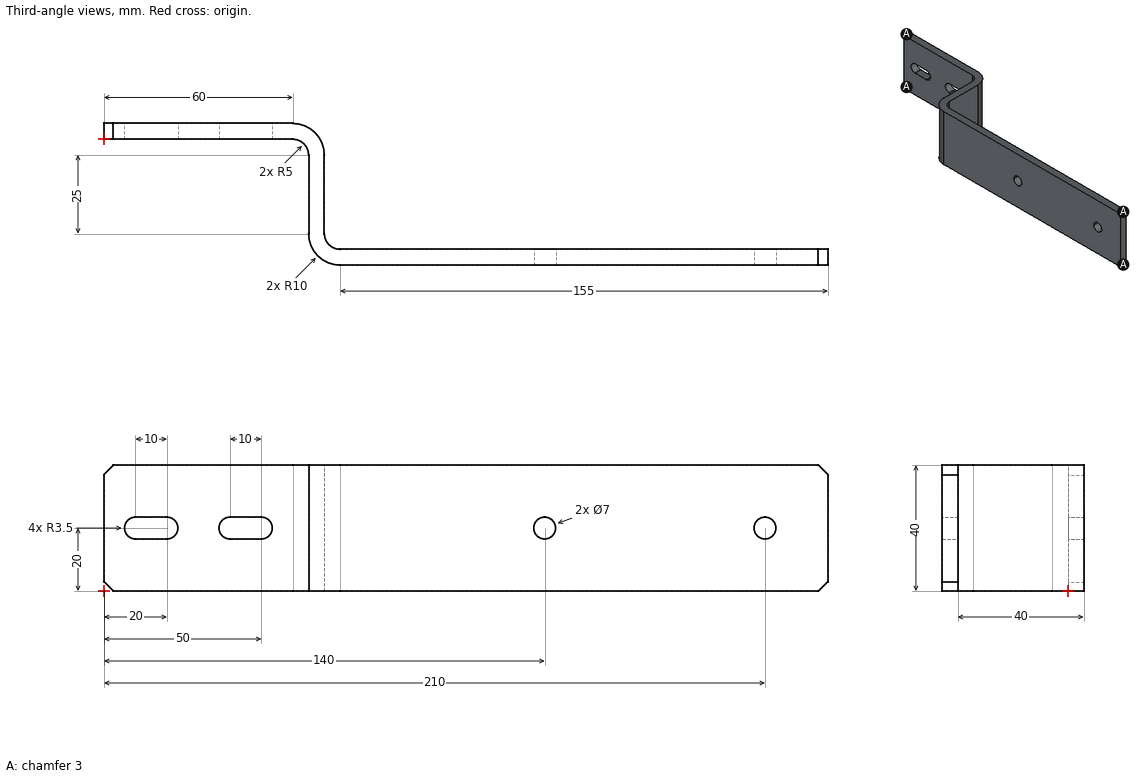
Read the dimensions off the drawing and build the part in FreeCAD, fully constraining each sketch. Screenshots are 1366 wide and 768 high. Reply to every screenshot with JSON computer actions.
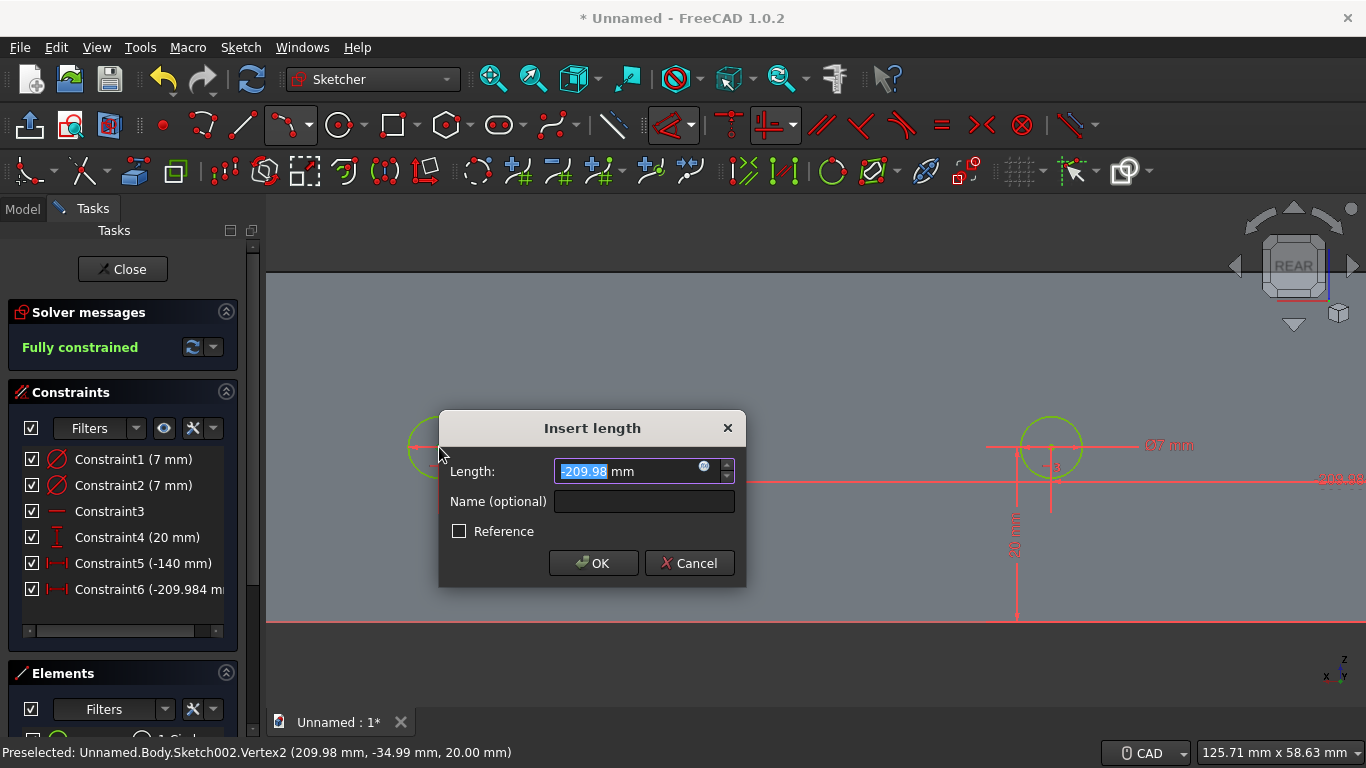
{"action": "type", "text": "-210"}
{"action": "key", "text": "Return"}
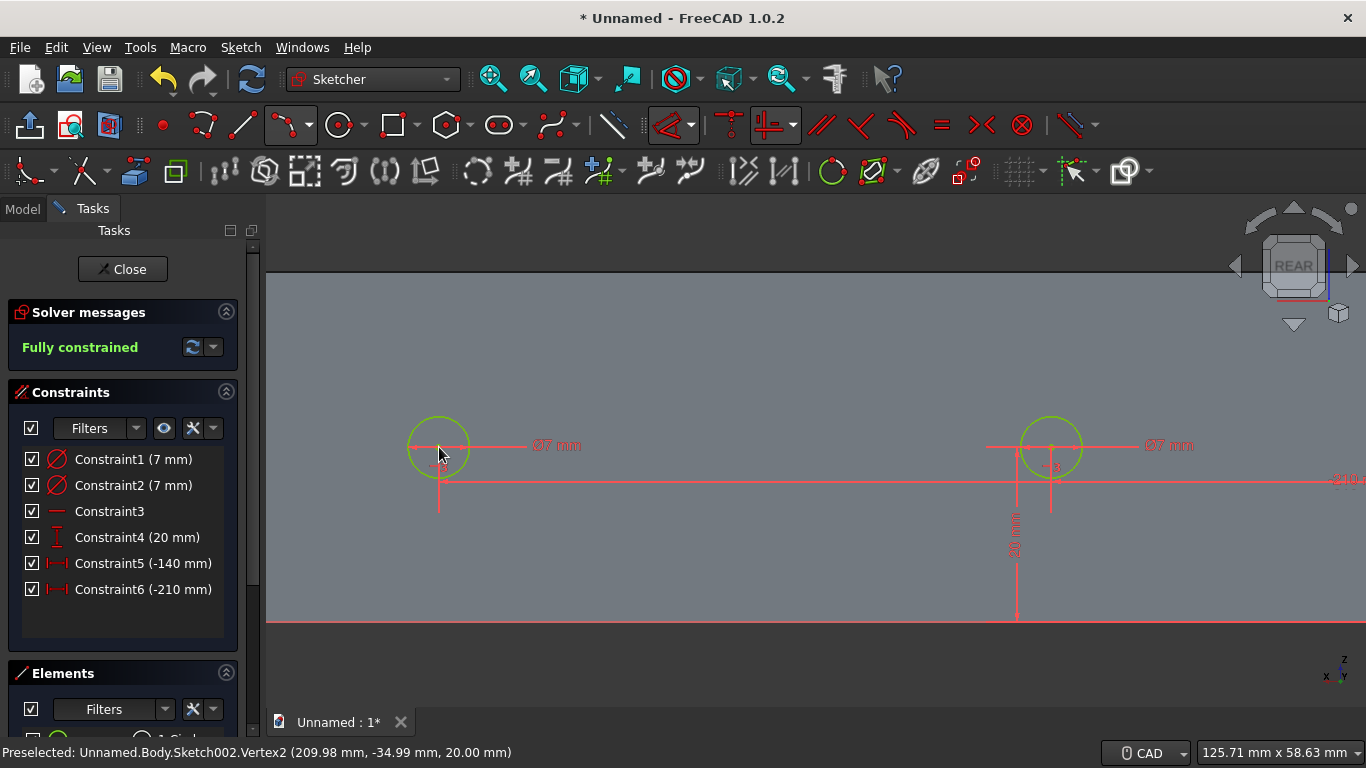
{"action": "left_click", "coordinate": [123, 269]}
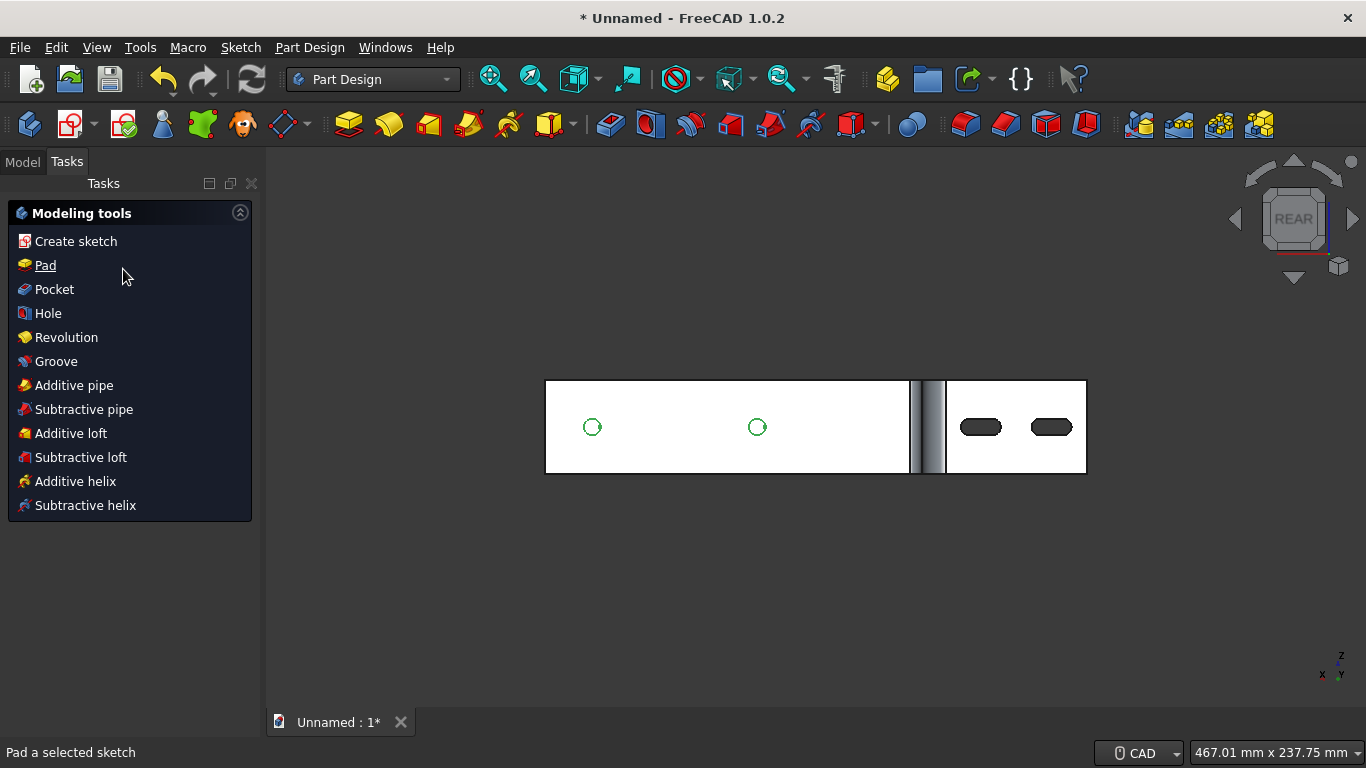
{"action": "left_click", "coordinate": [612, 124]}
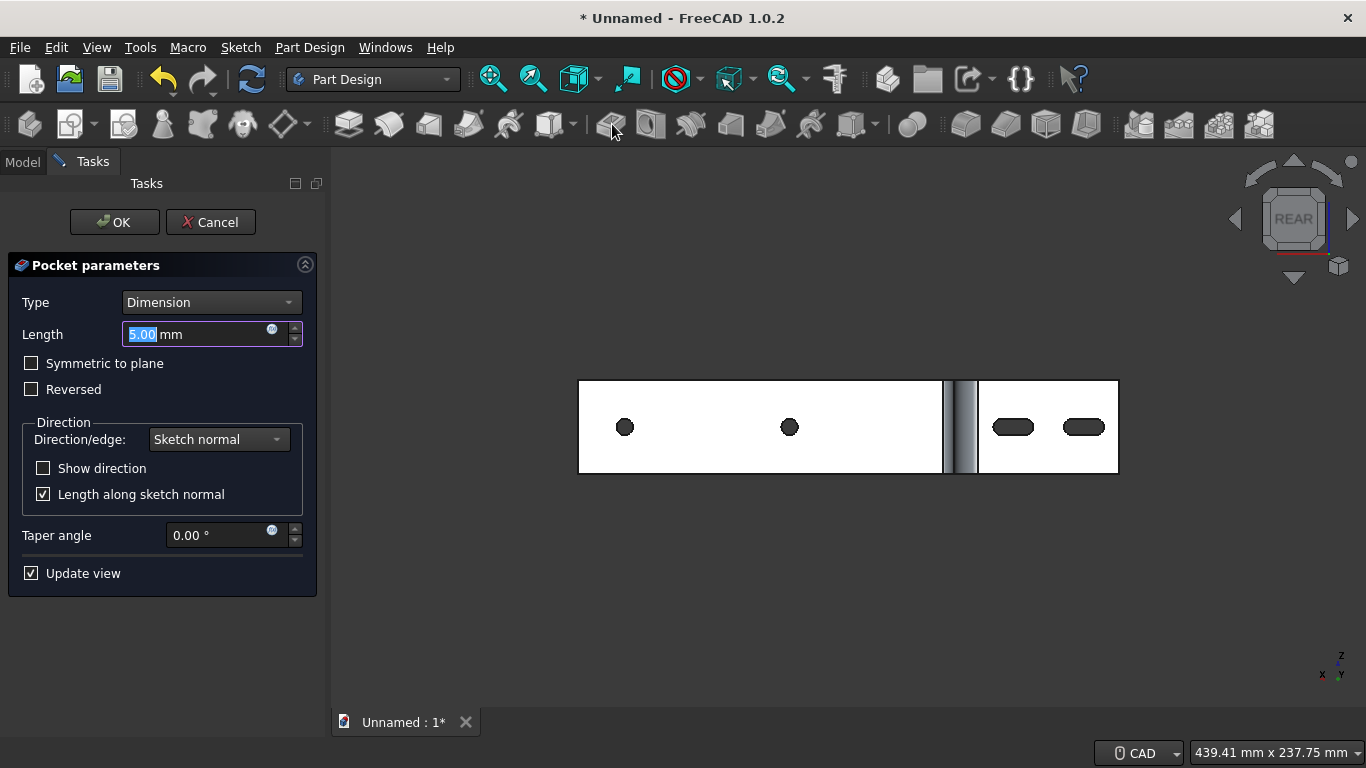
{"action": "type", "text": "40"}
{"action": "key", "text": "Tab"}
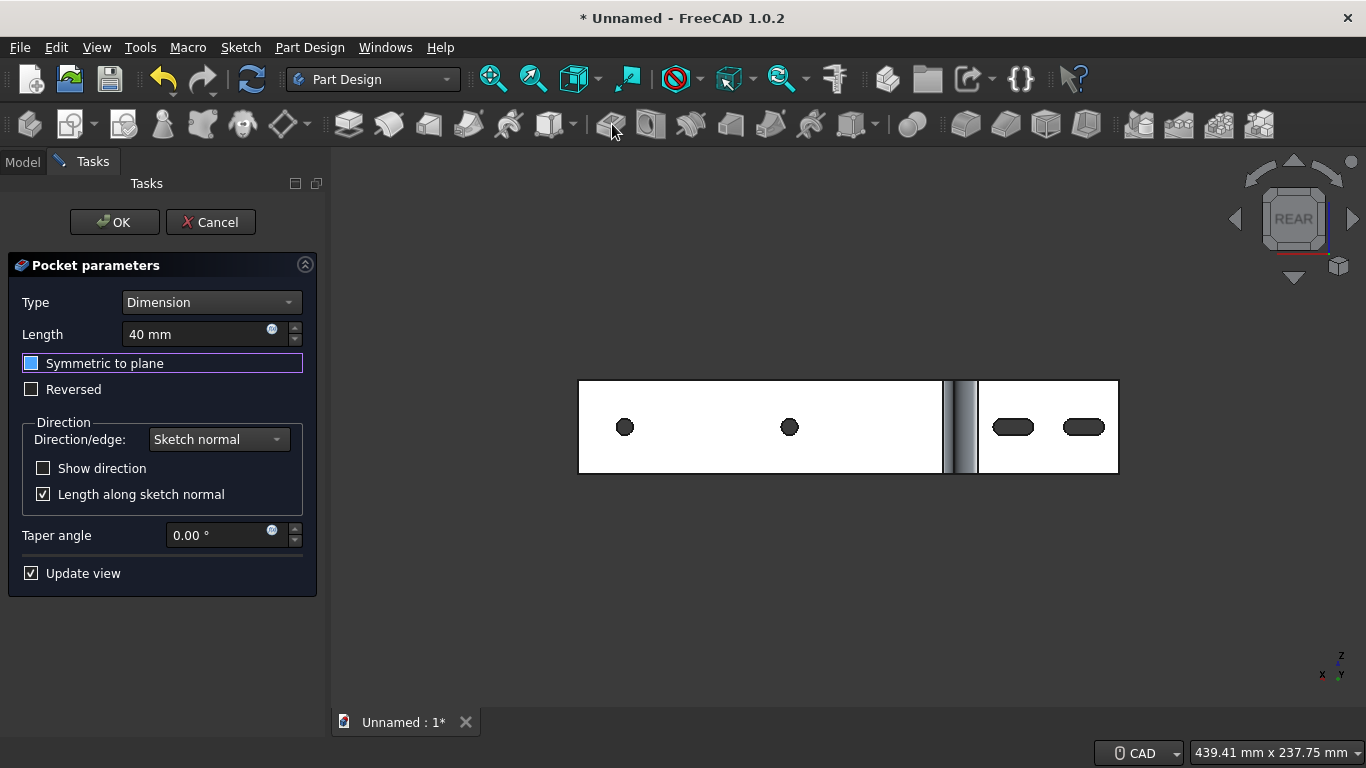
{"action": "left_click", "coordinate": [115, 222]}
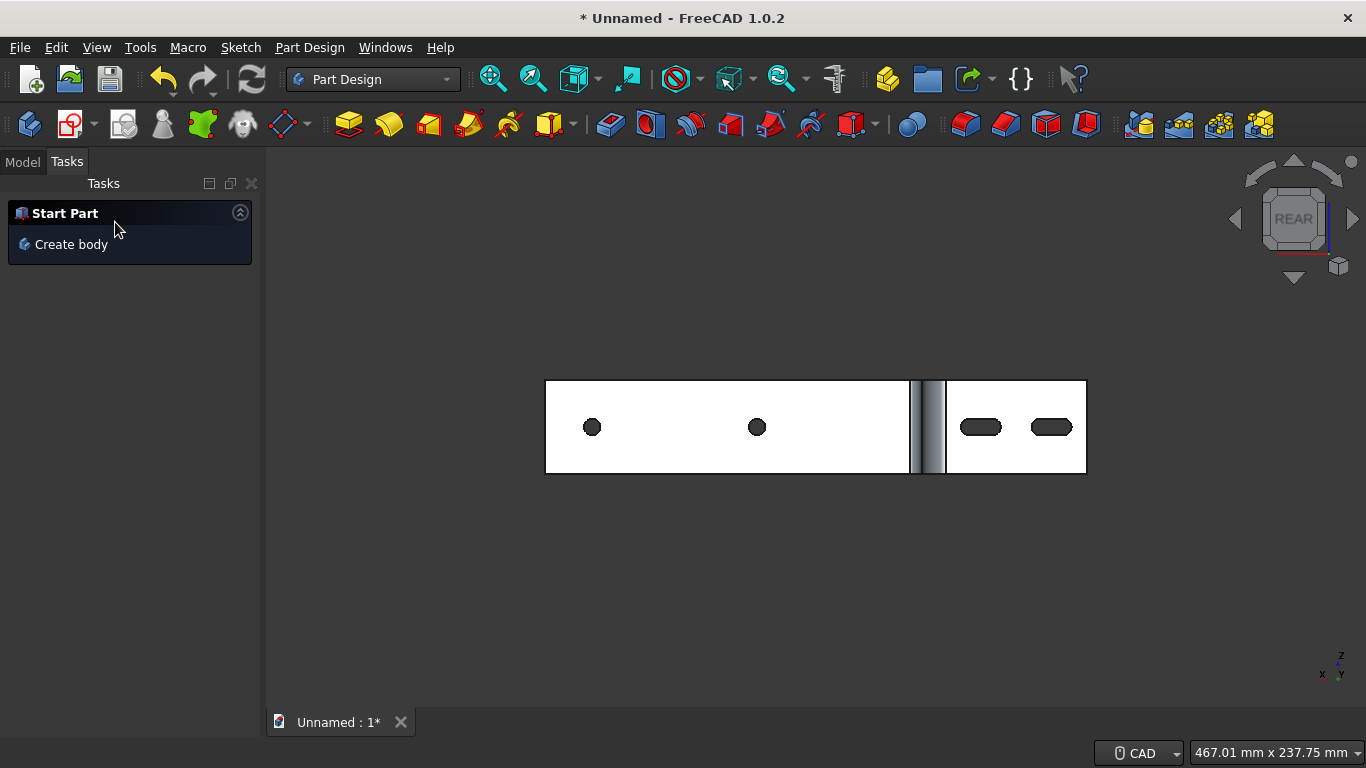
{"action": "scroll", "coordinate": [1087, 473], "scroll_direction": "up", "scroll_amount": 7}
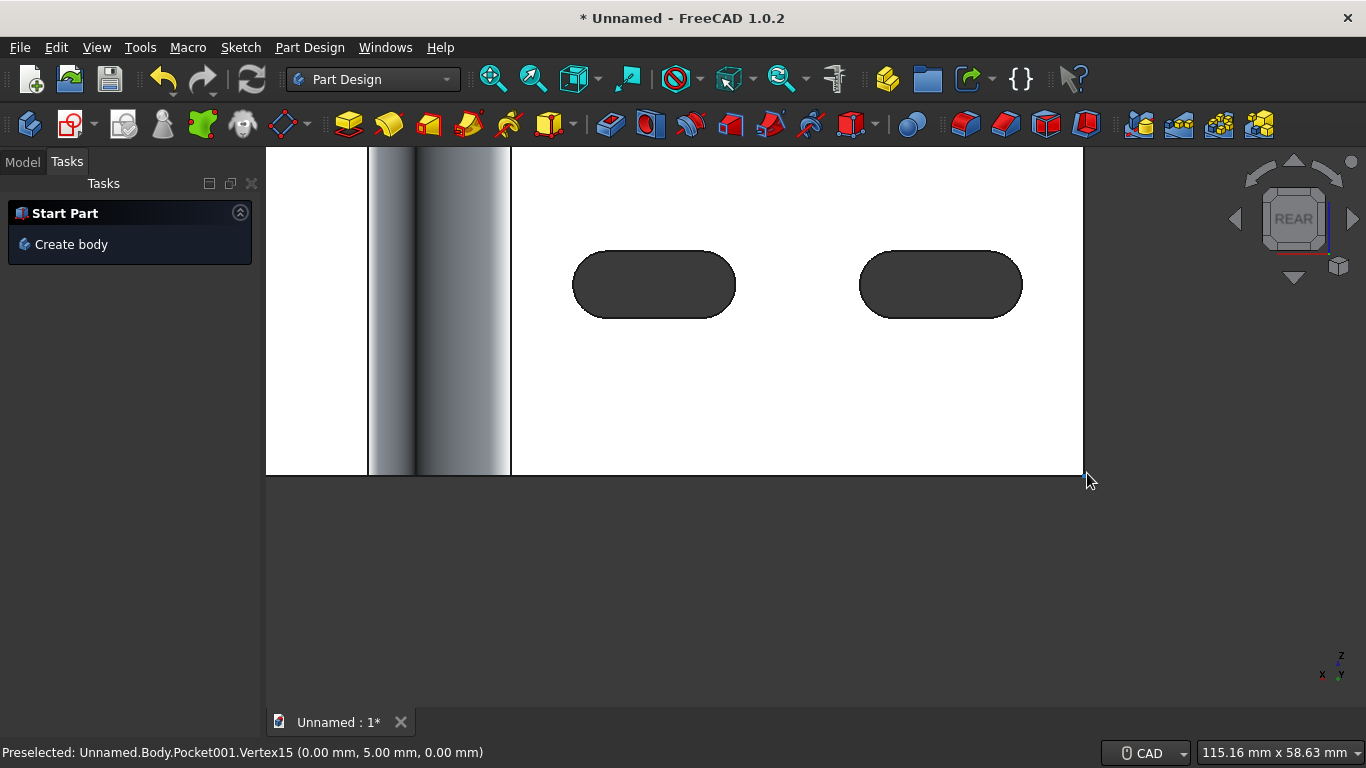
{"action": "left_click", "coordinate": [494, 80]}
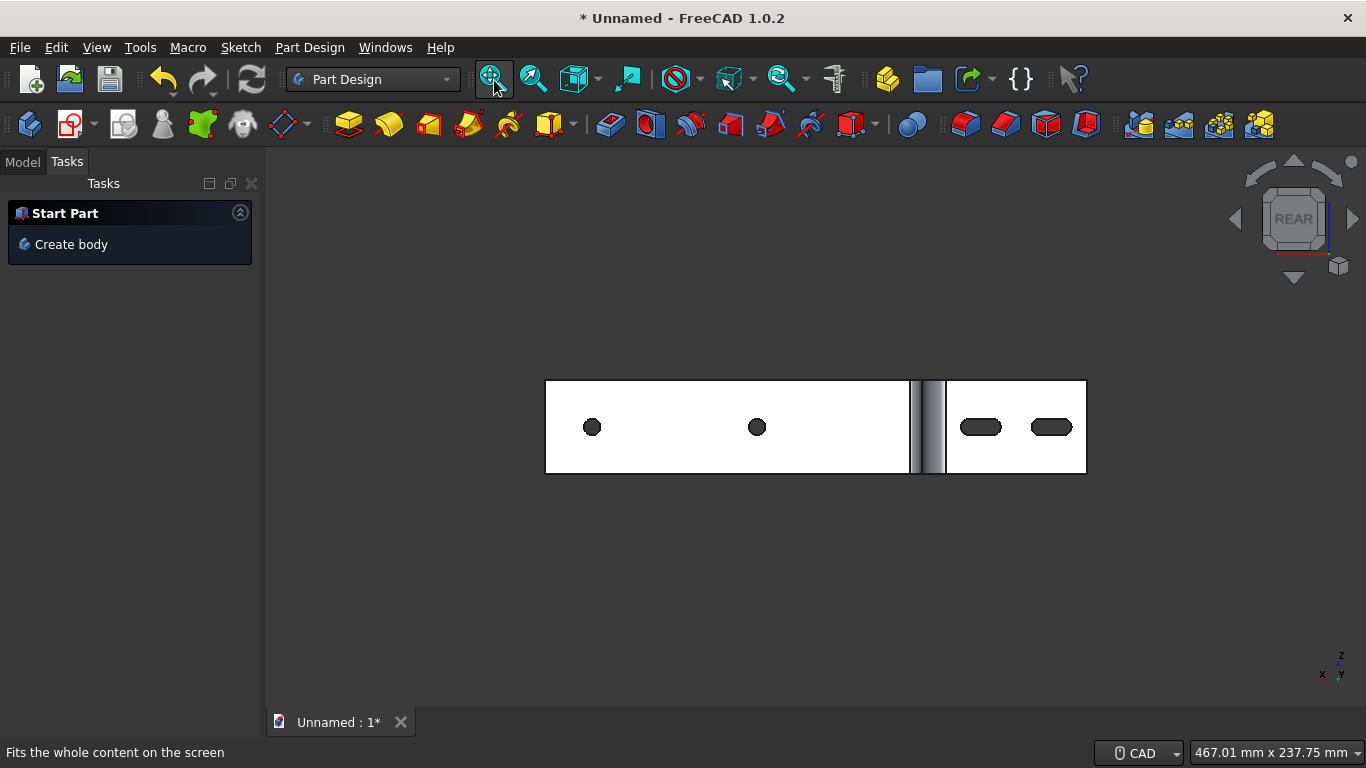
{"action": "key", "text": "0"}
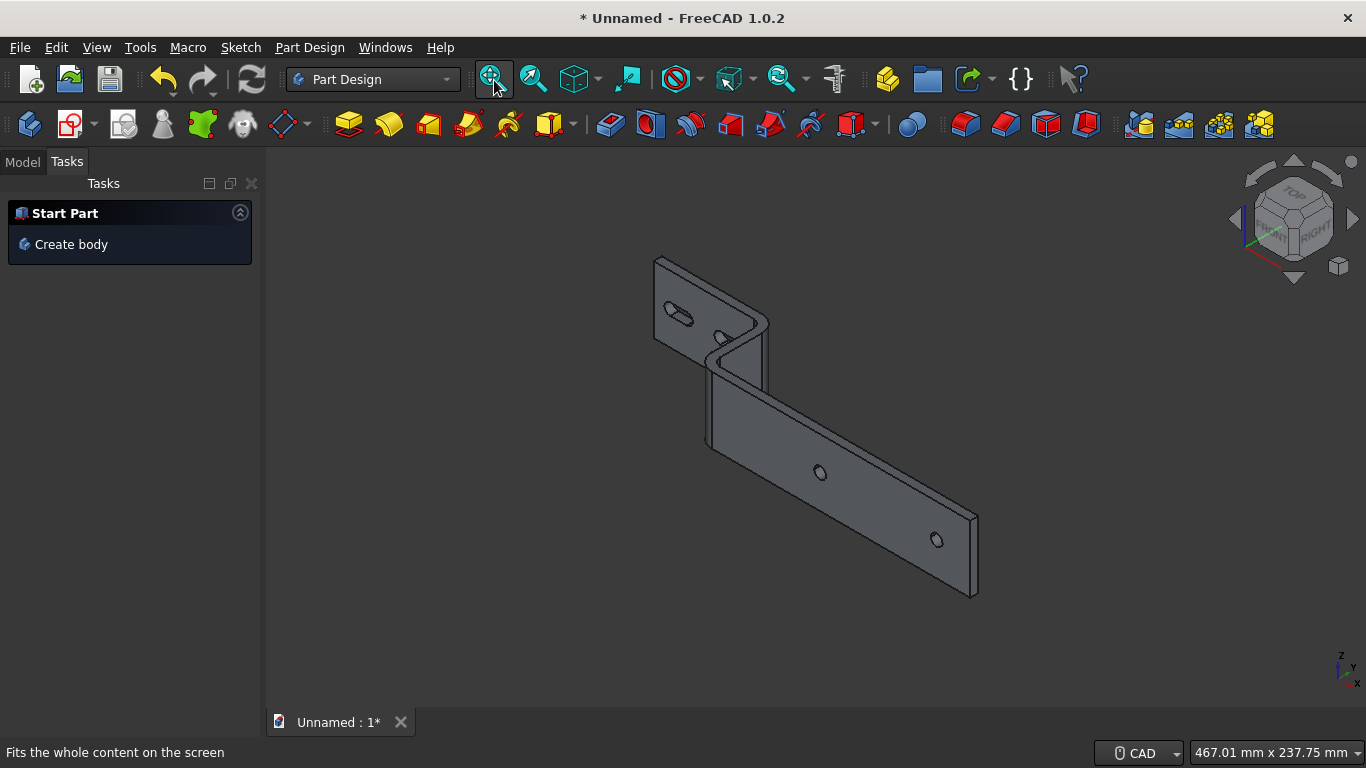
{"action": "left_click", "coordinate": [976, 516]}